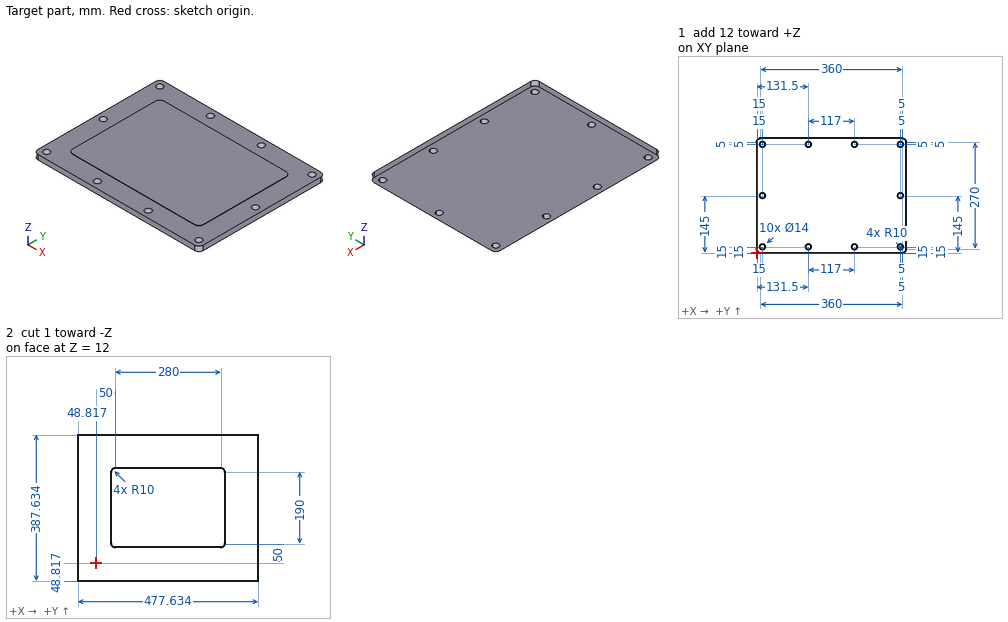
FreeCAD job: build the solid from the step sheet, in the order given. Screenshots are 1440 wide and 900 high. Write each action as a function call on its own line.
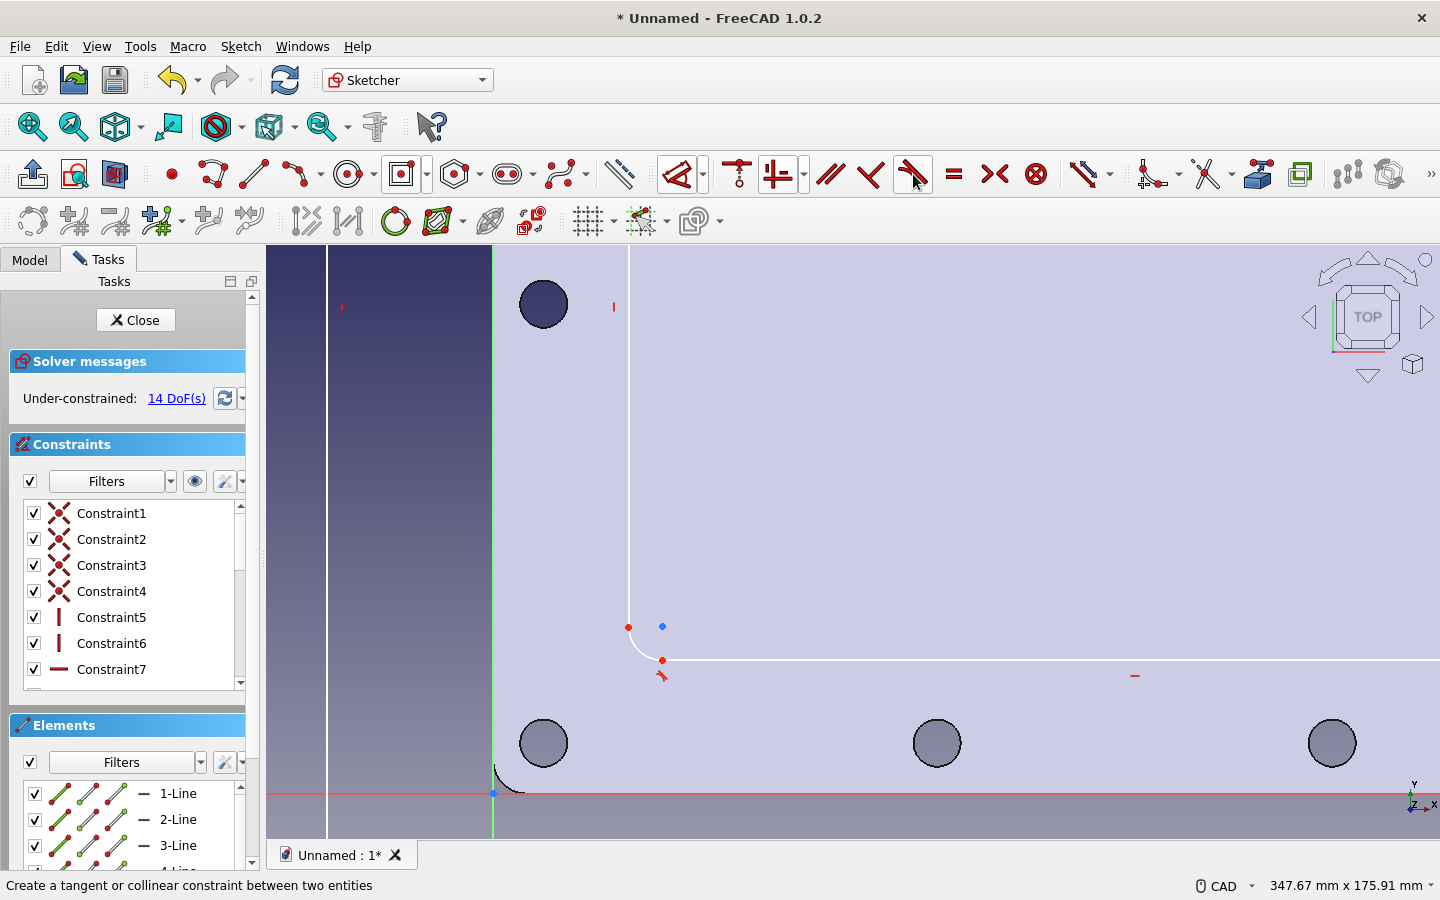
click(629, 435)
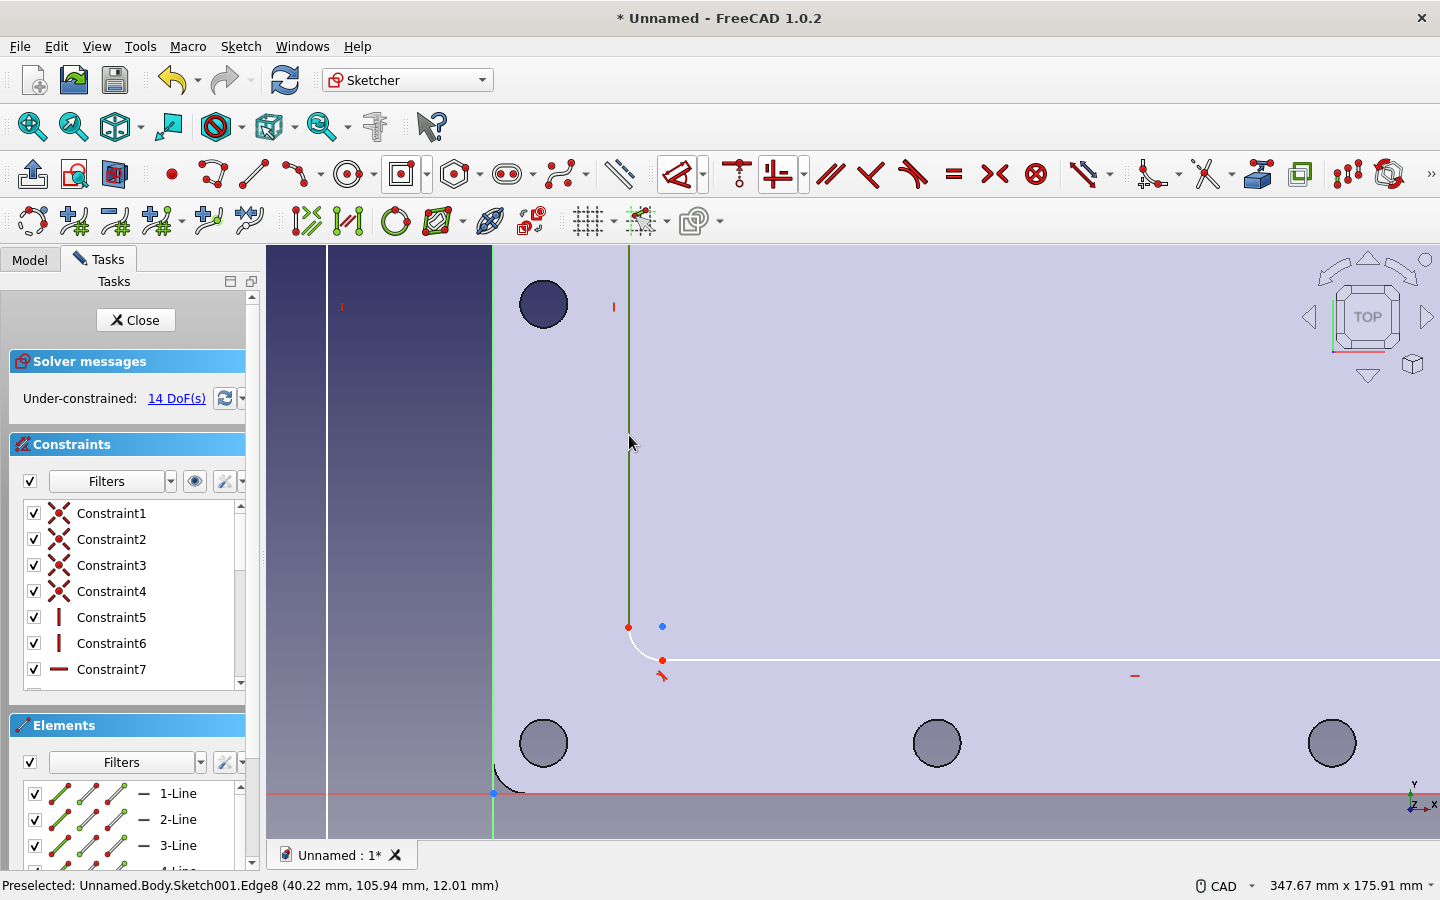
click(633, 643)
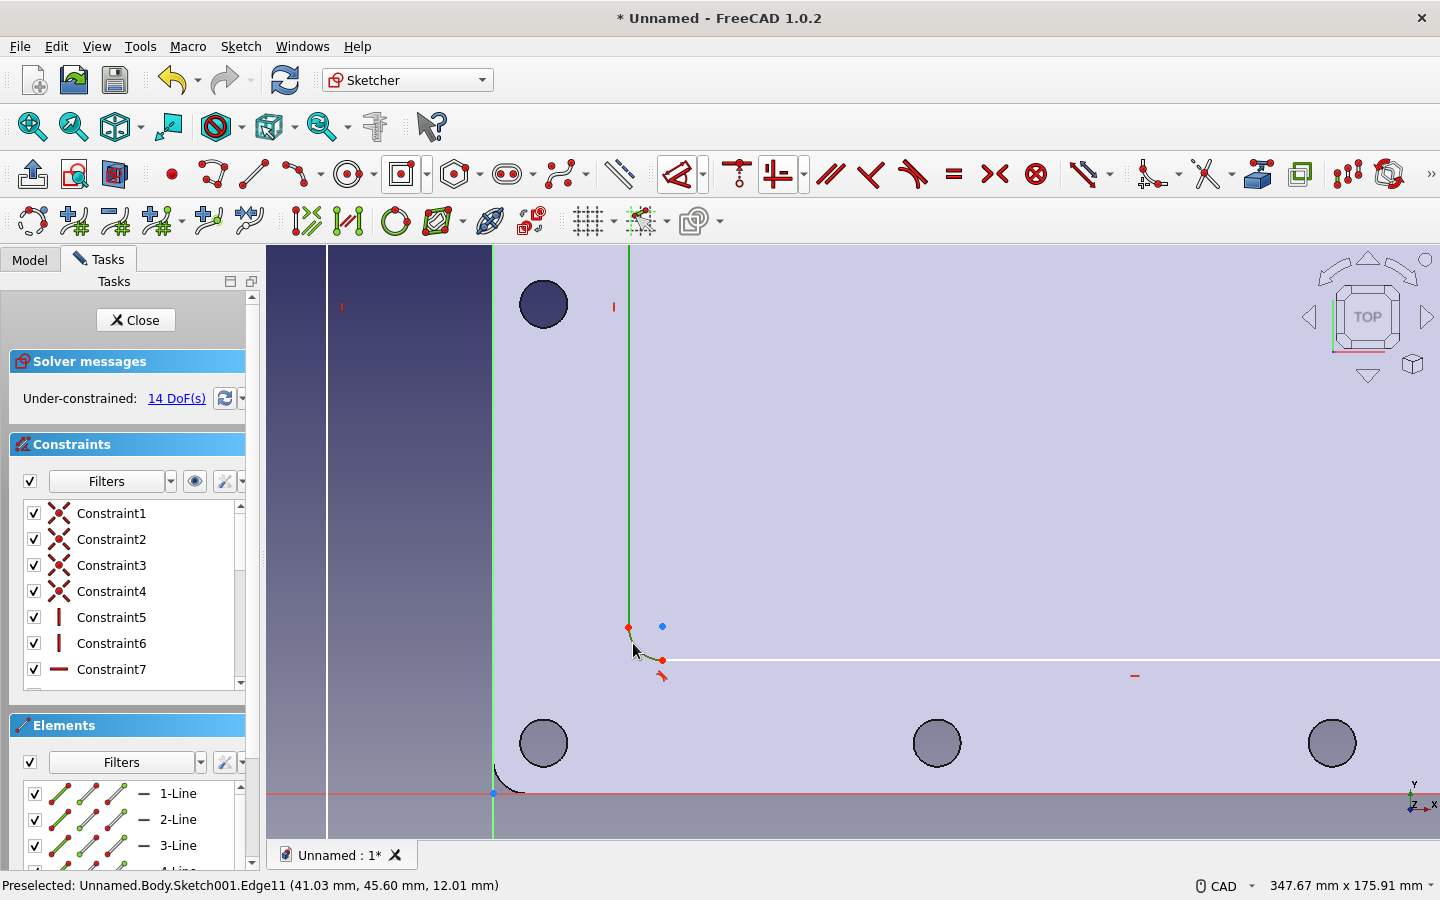
click(913, 174)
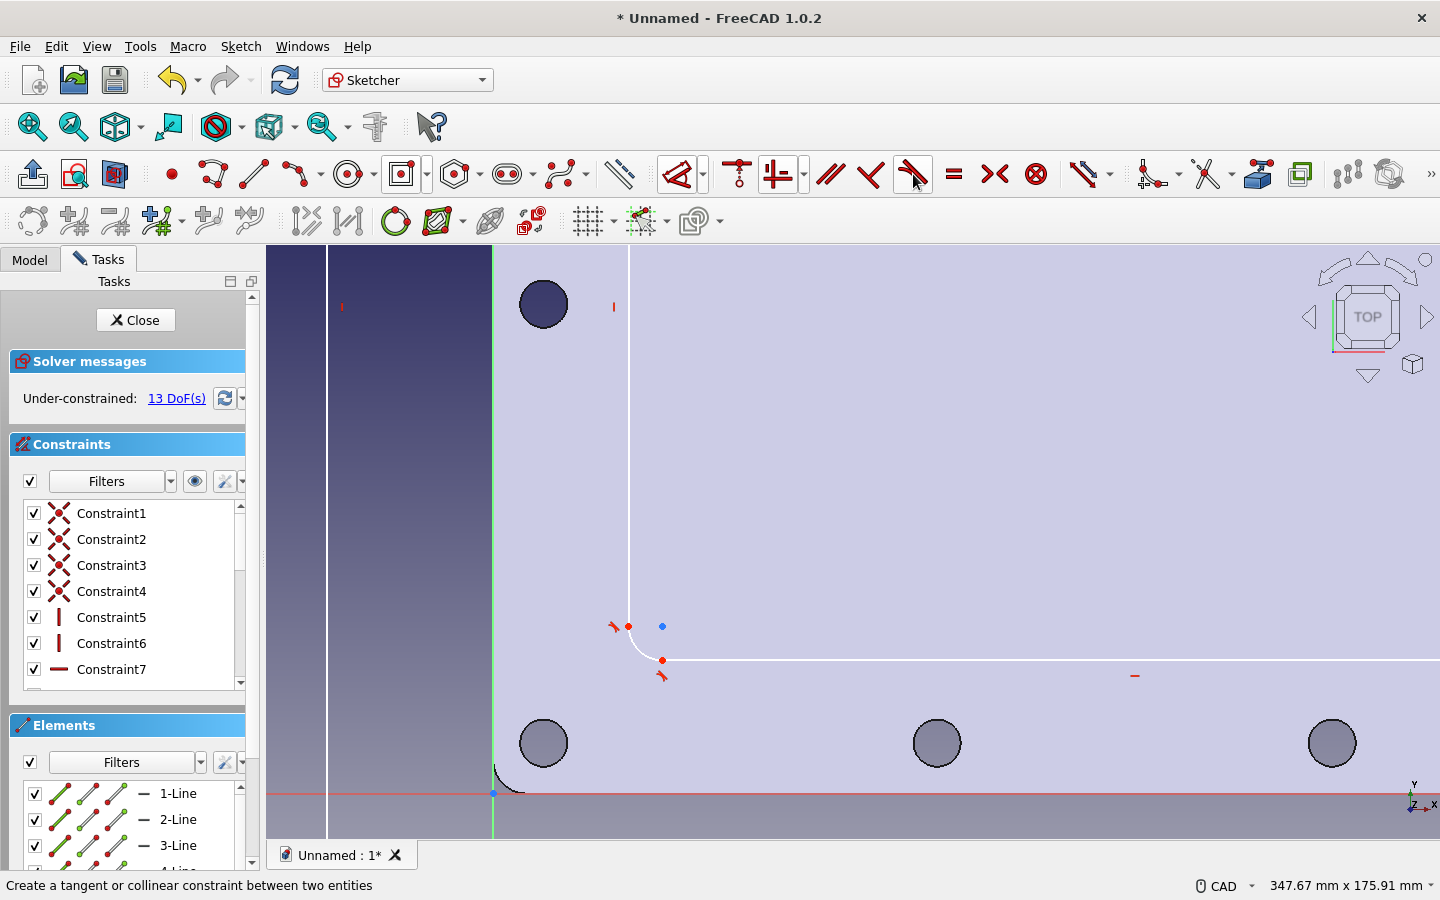
click(629, 434)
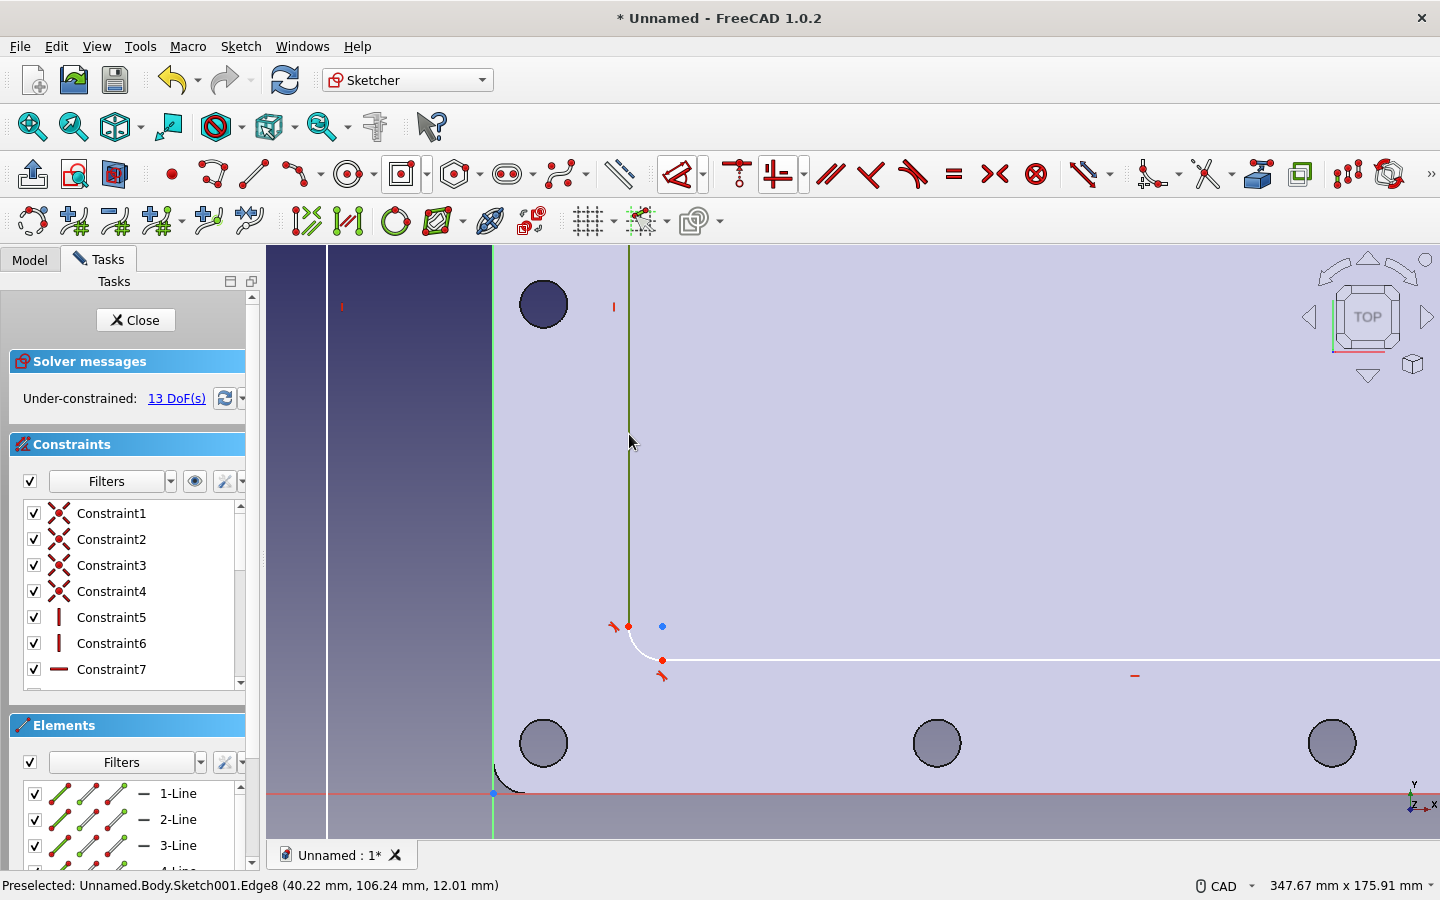
scroll(634, 645, down, 6)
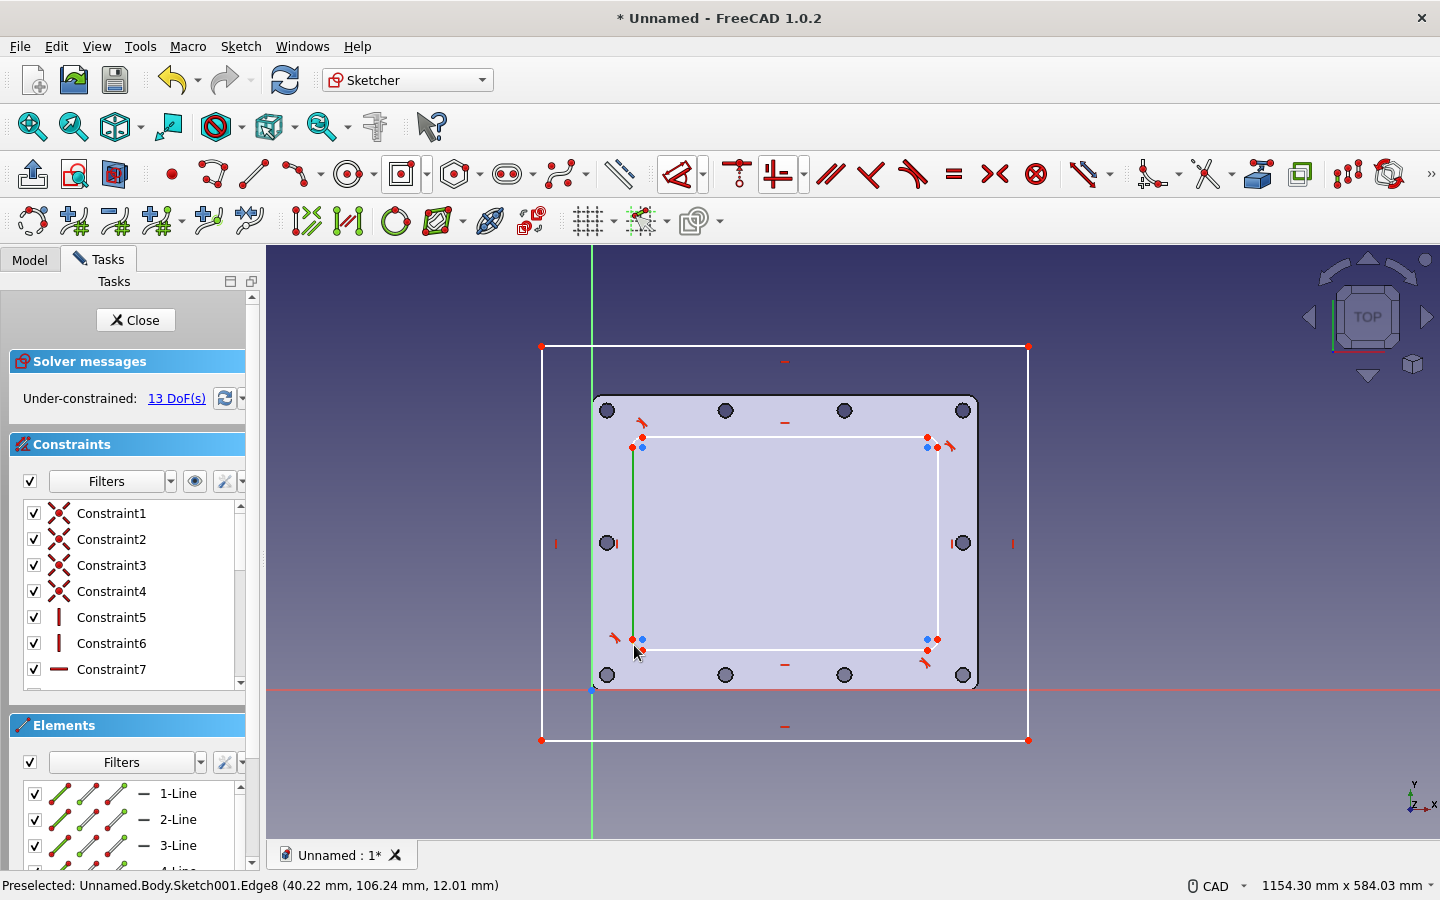
scroll(638, 438, up, 6)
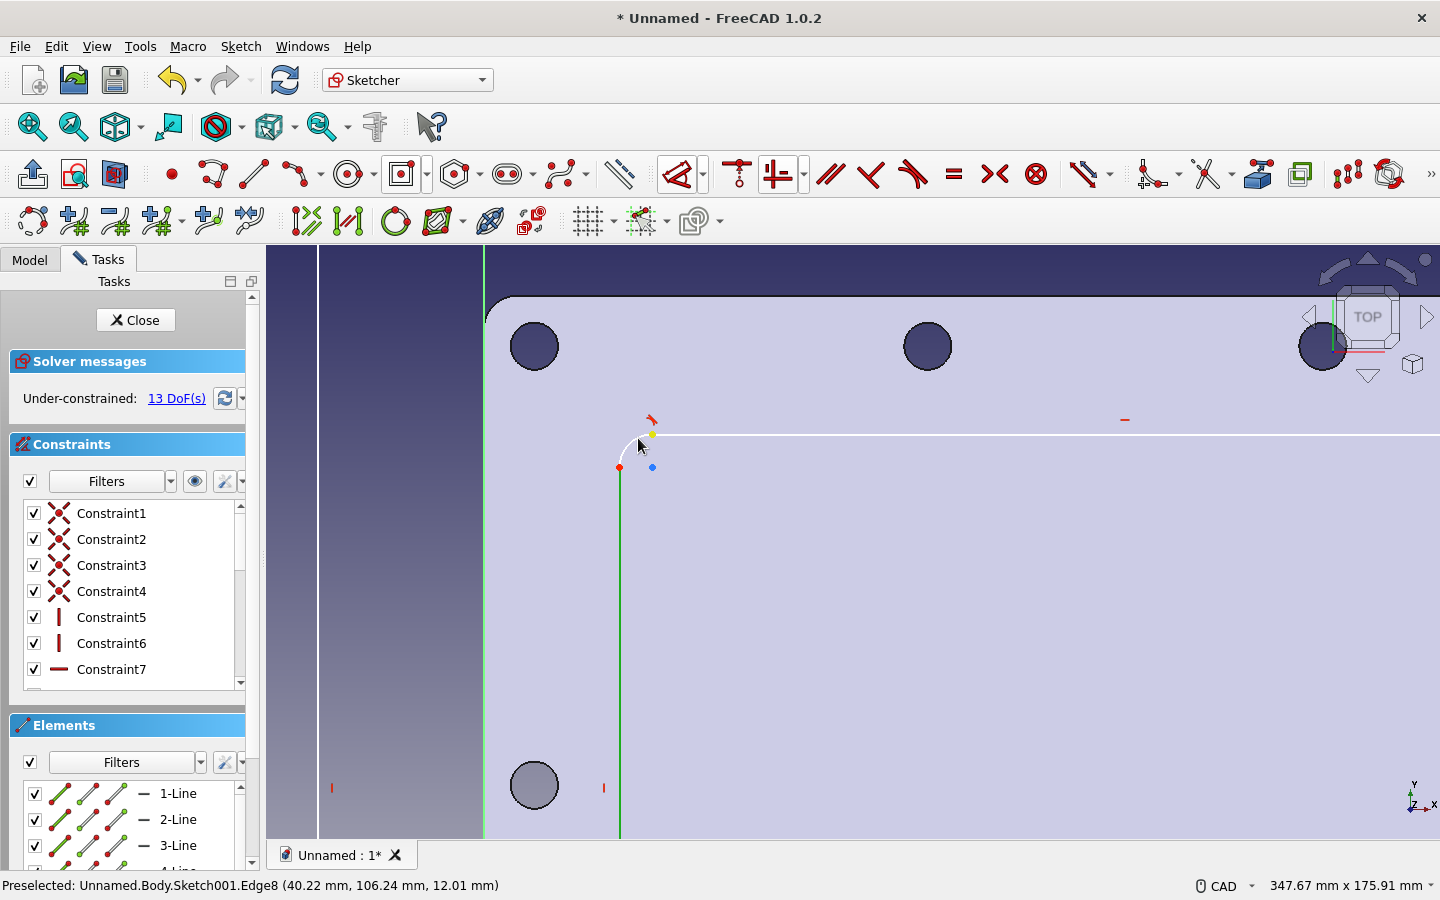
click(638, 438)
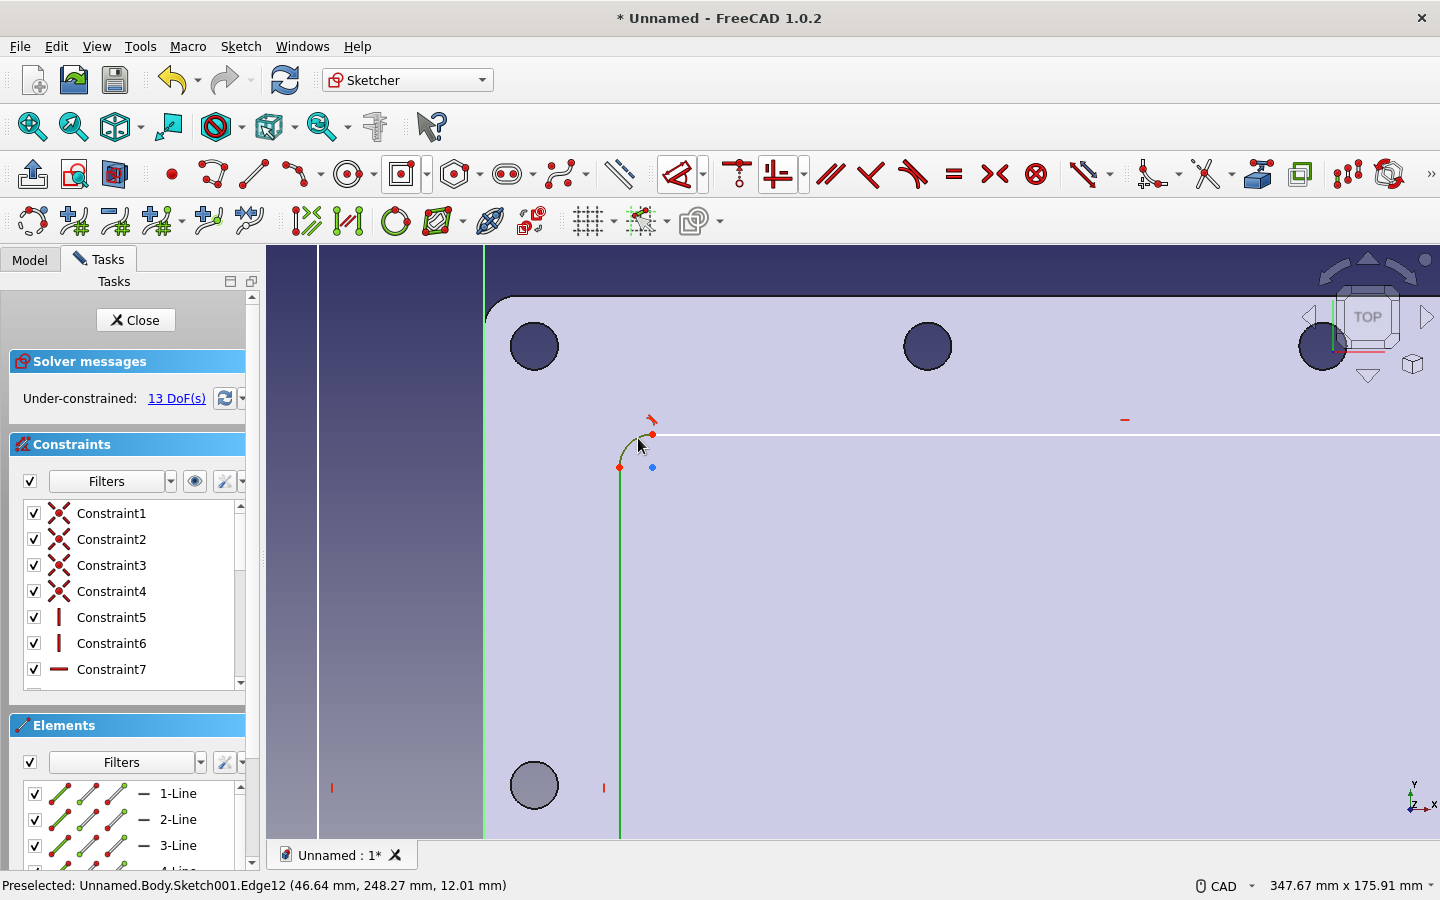
click(913, 174)